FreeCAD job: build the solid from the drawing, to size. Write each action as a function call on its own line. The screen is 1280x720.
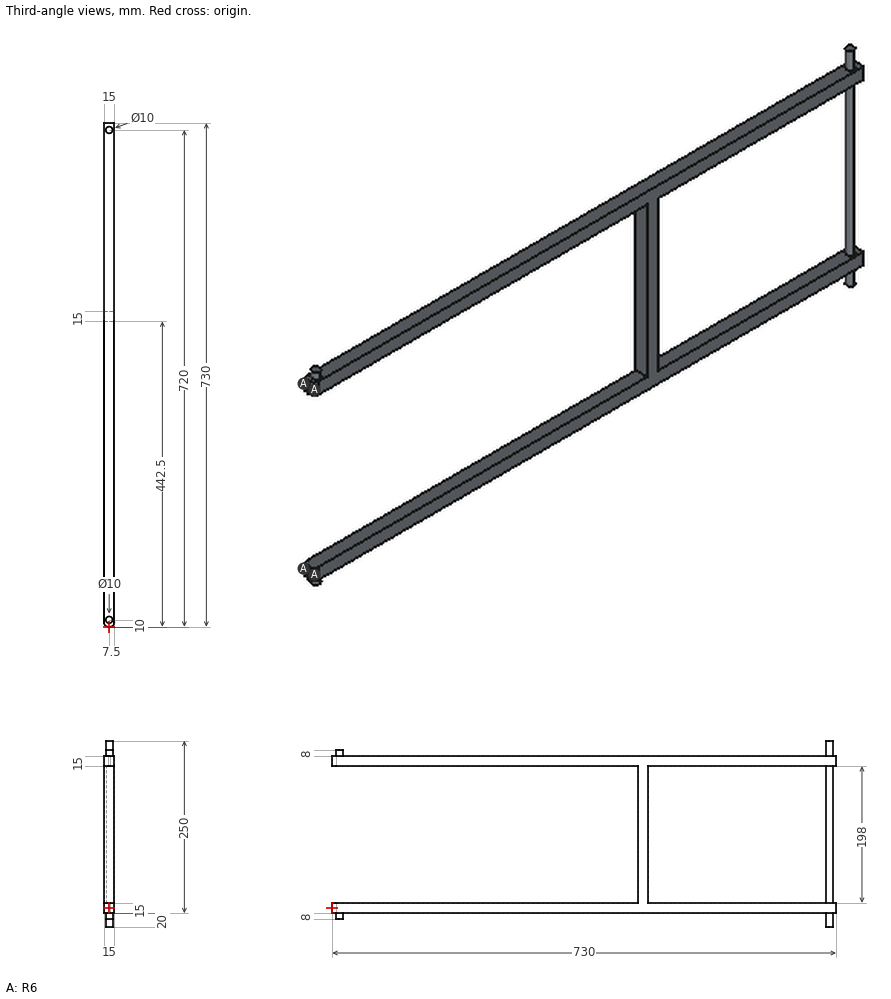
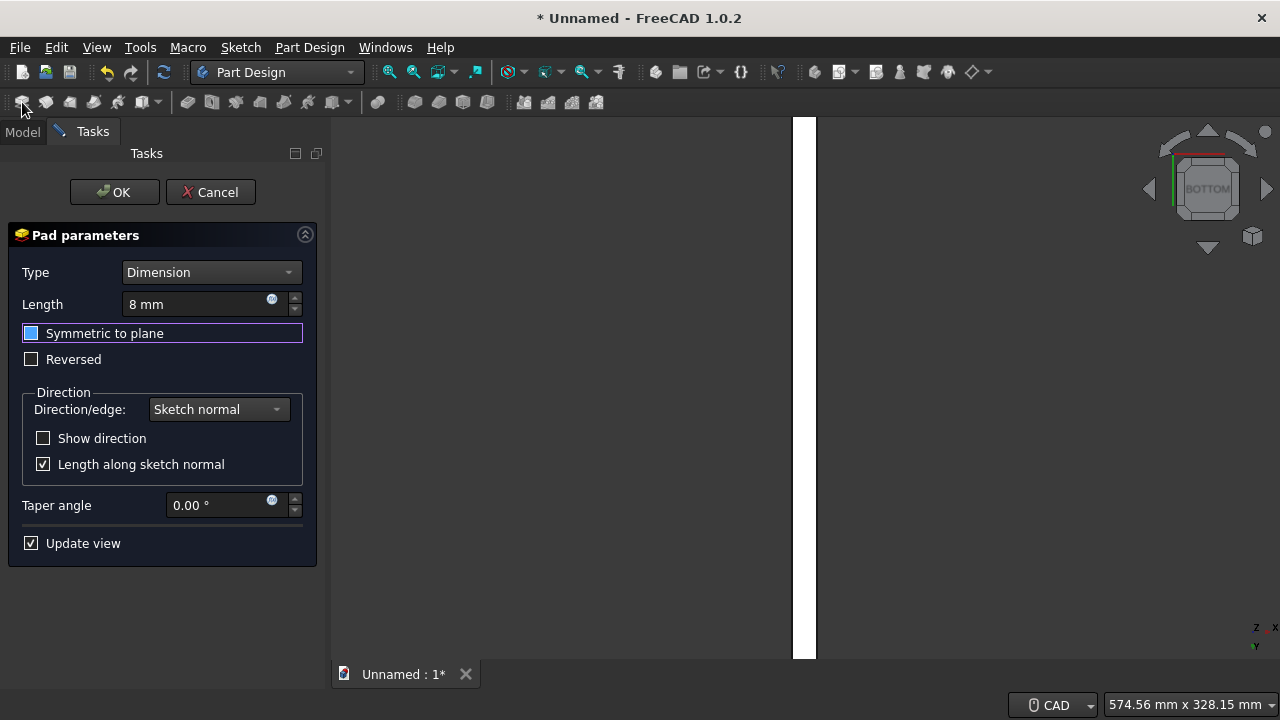
click(115, 192)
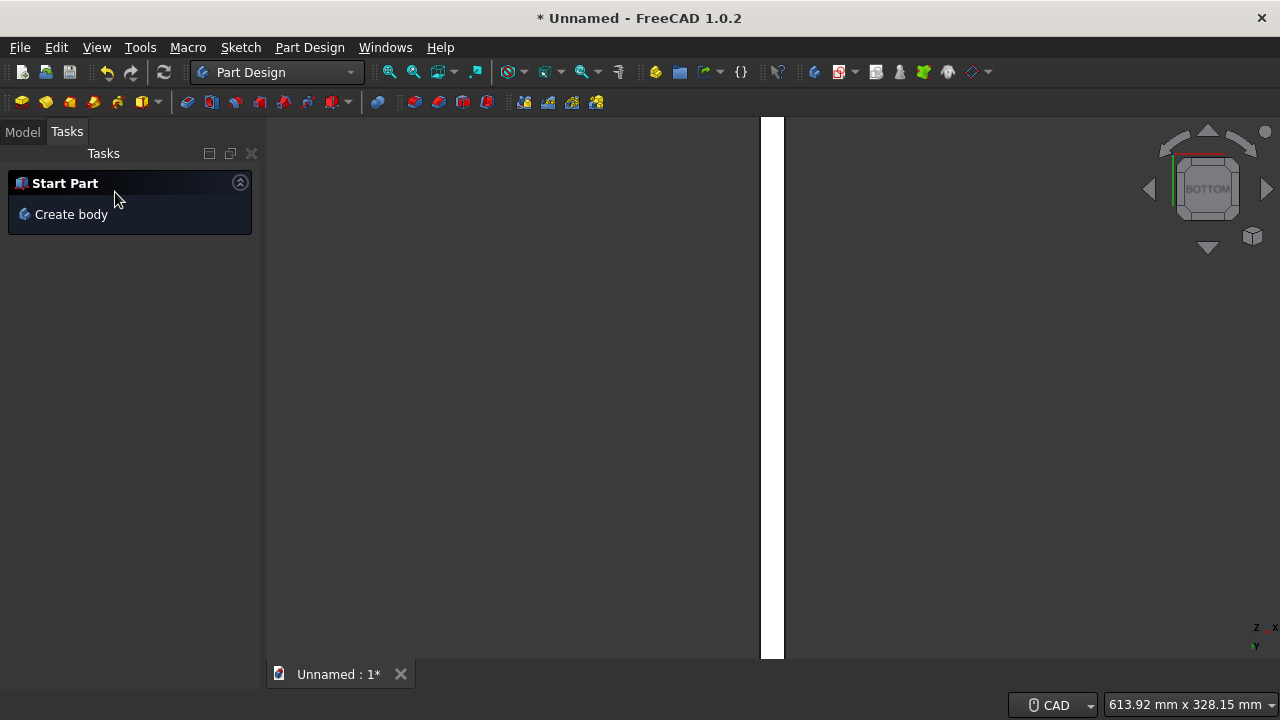
click(390, 72)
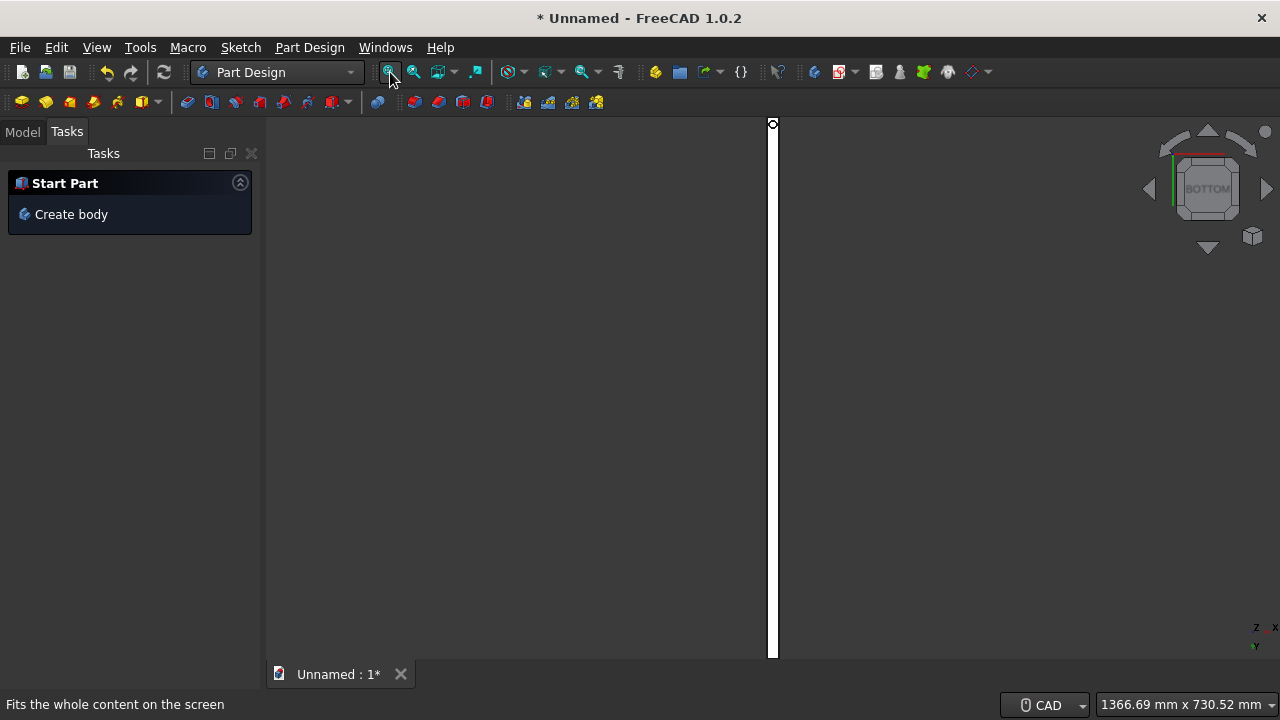
key(0)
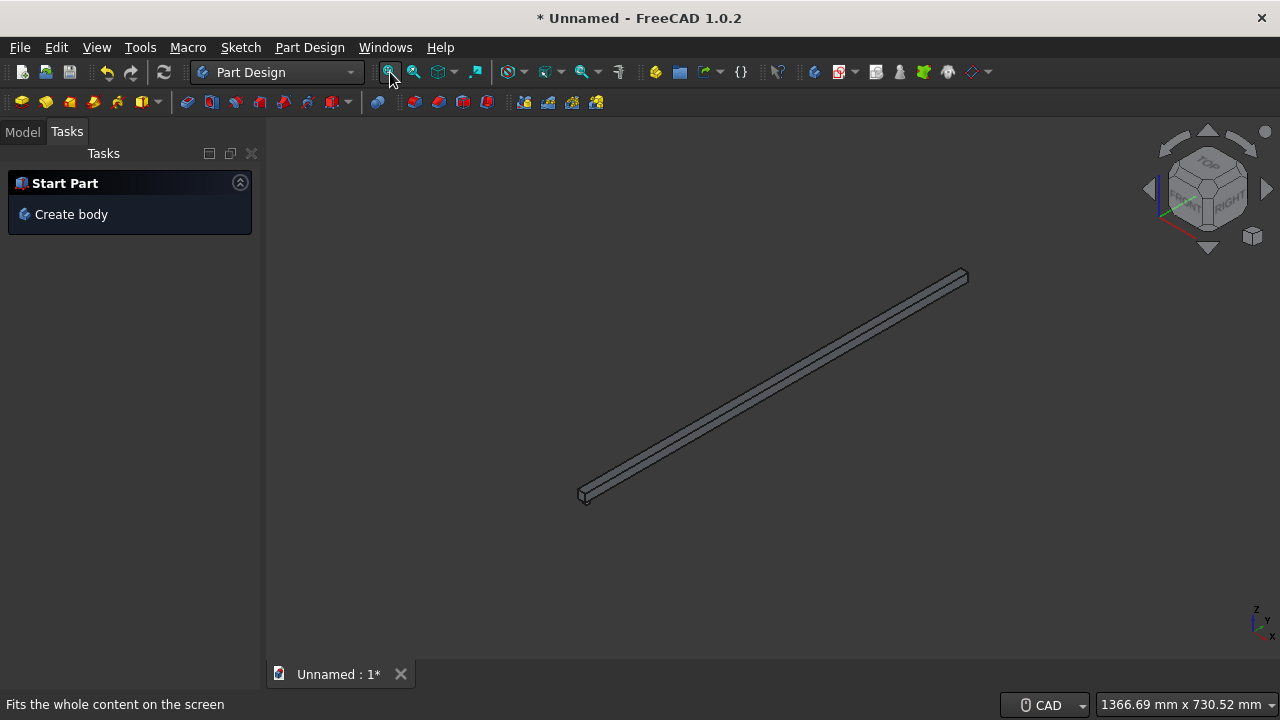
click(390, 72)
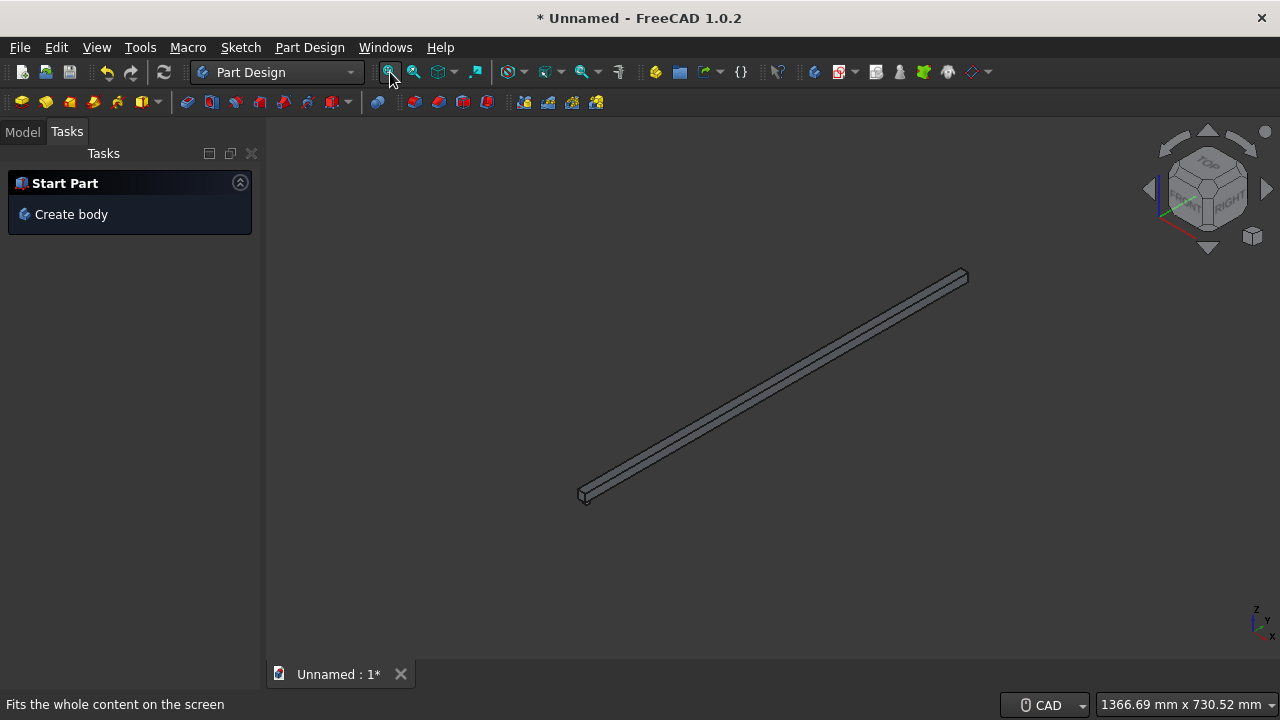
scroll(937, 285, up, 4)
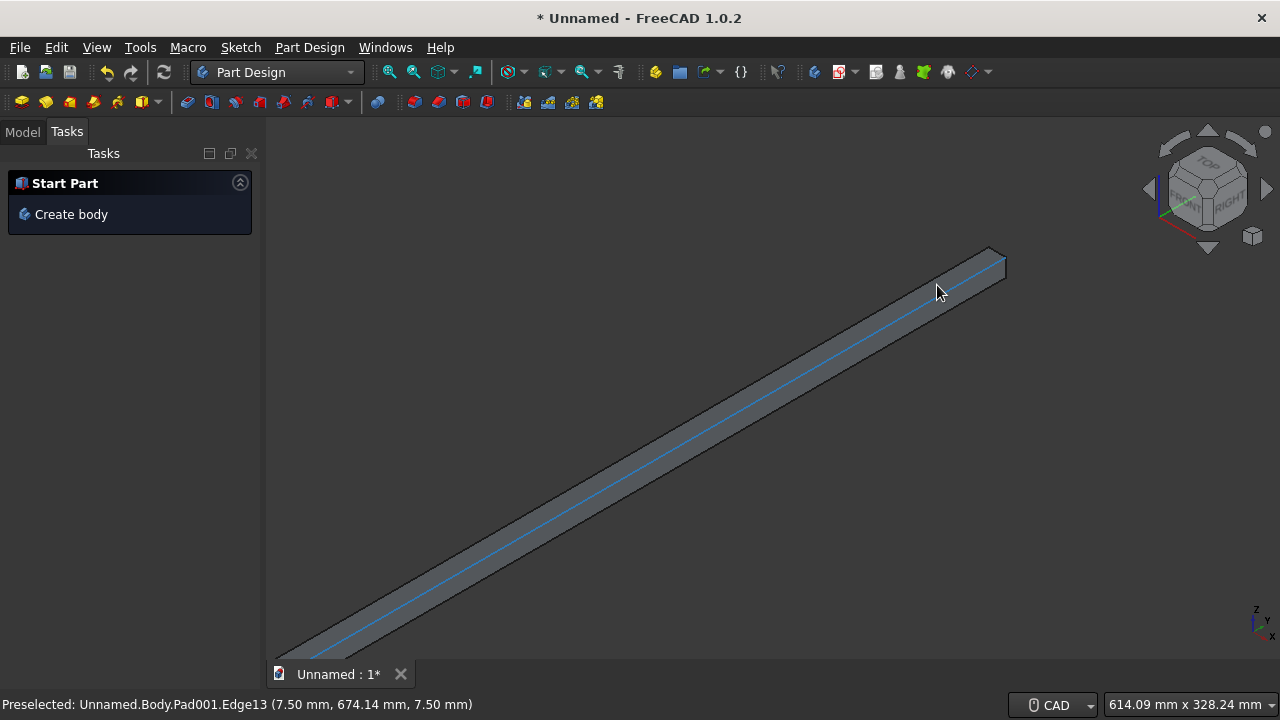
click(936, 286)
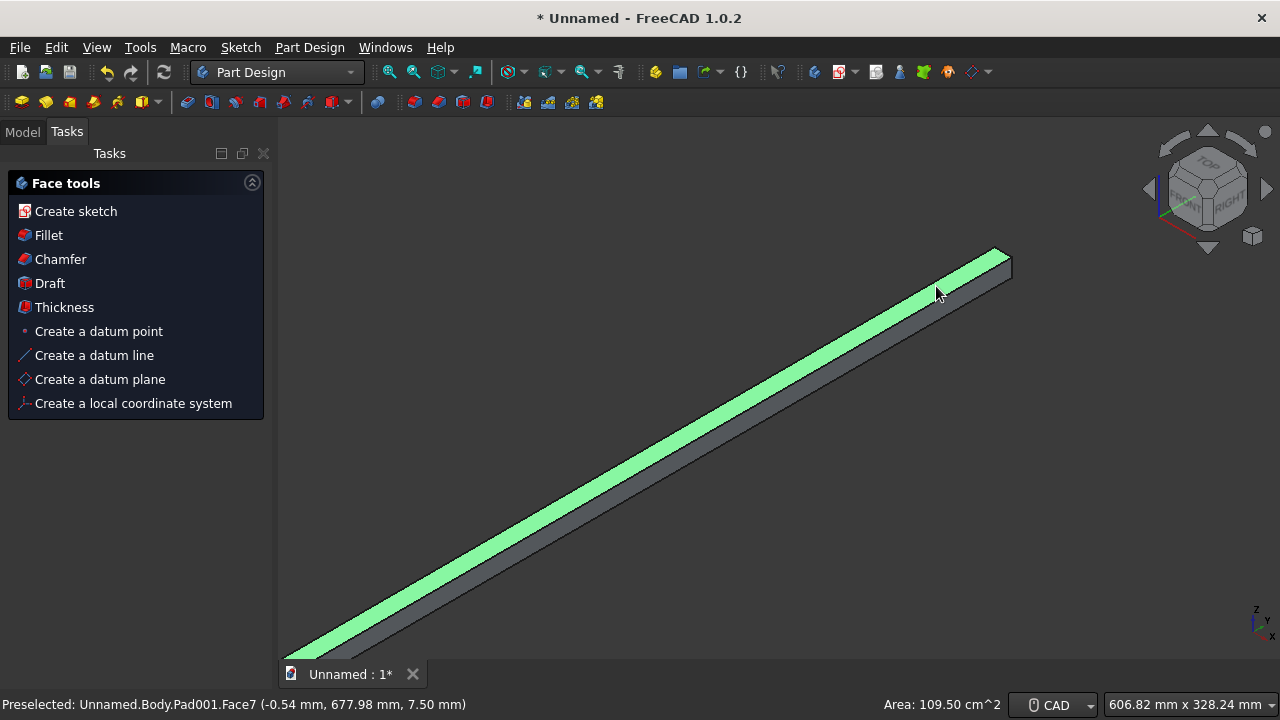
click(840, 72)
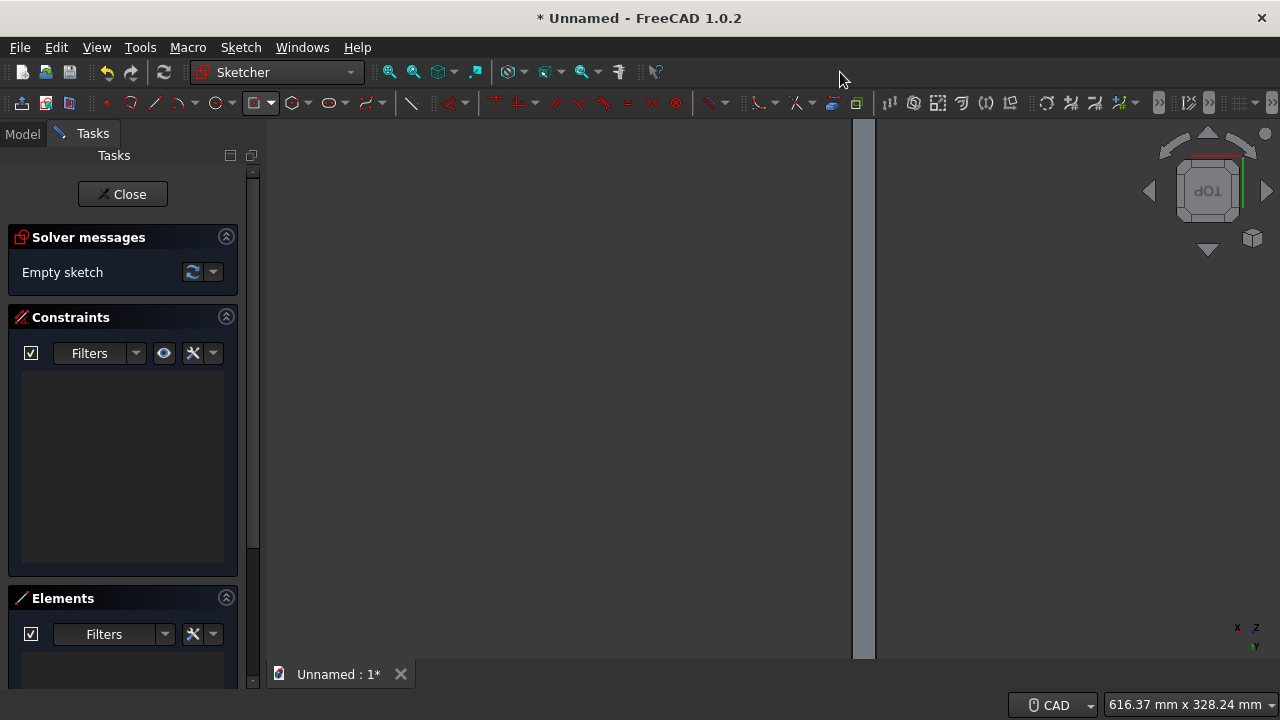
scroll(877, 331, up, 13)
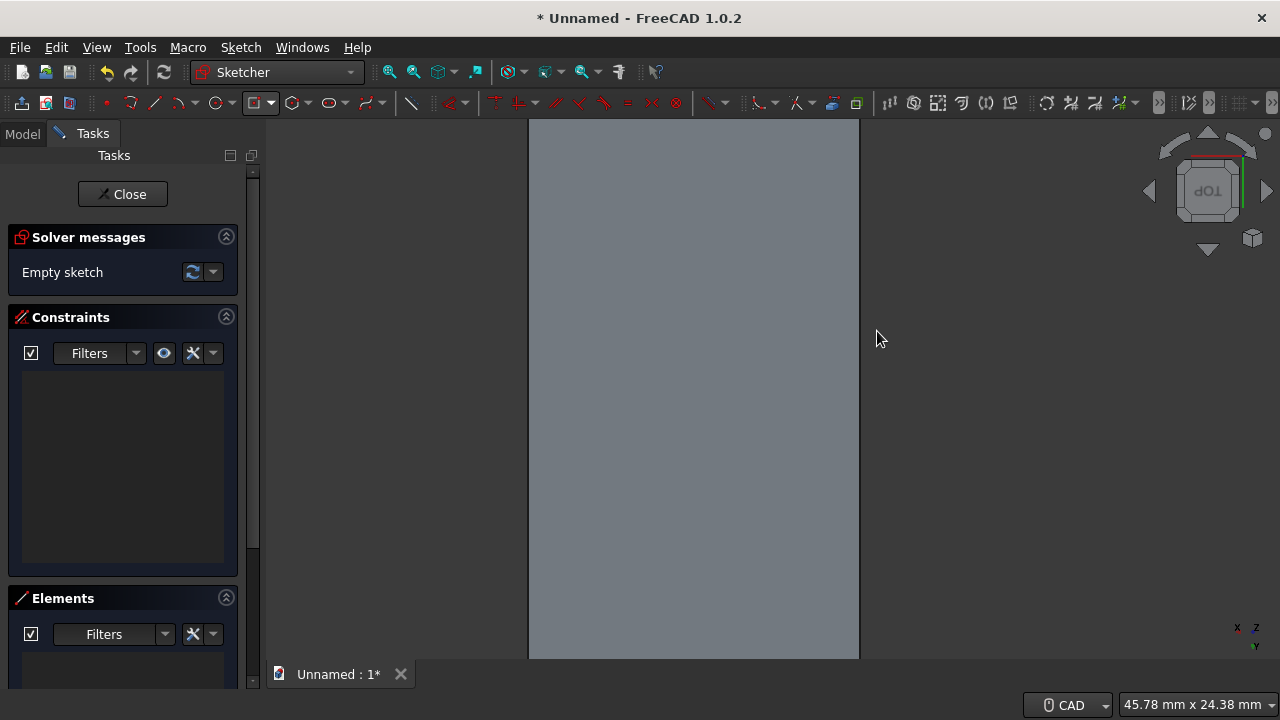
click(274, 104)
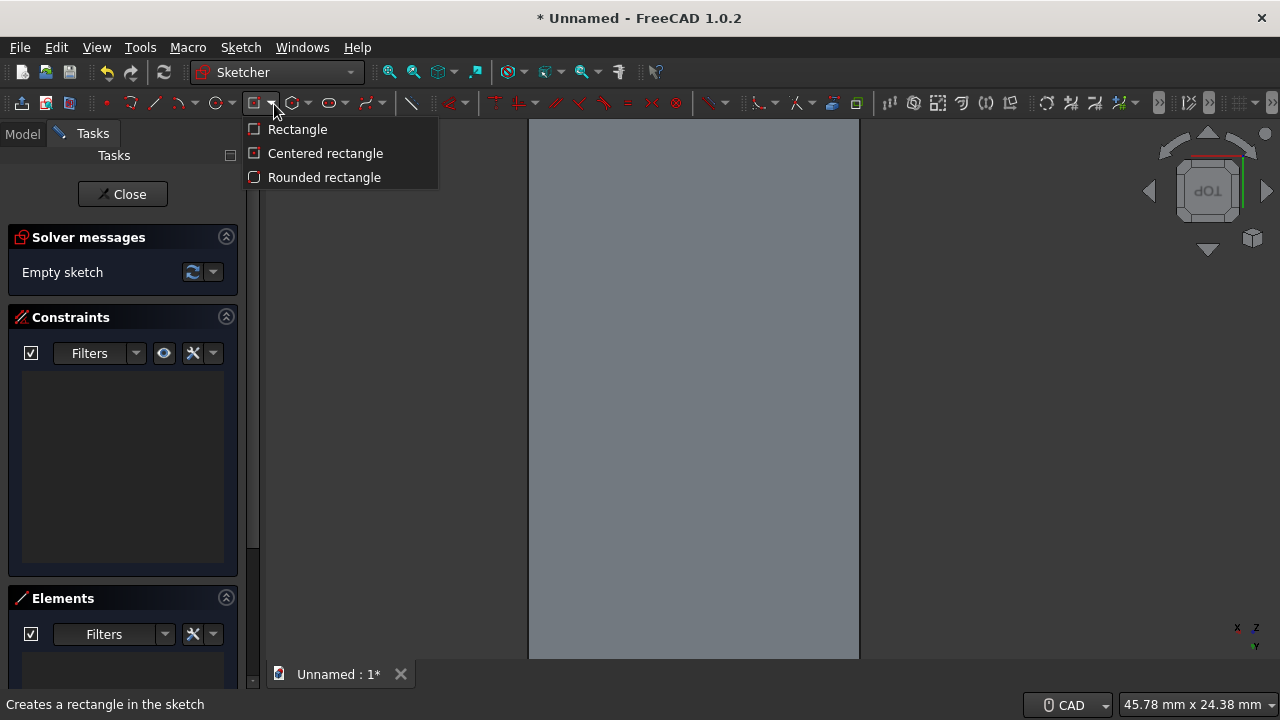
click(340, 129)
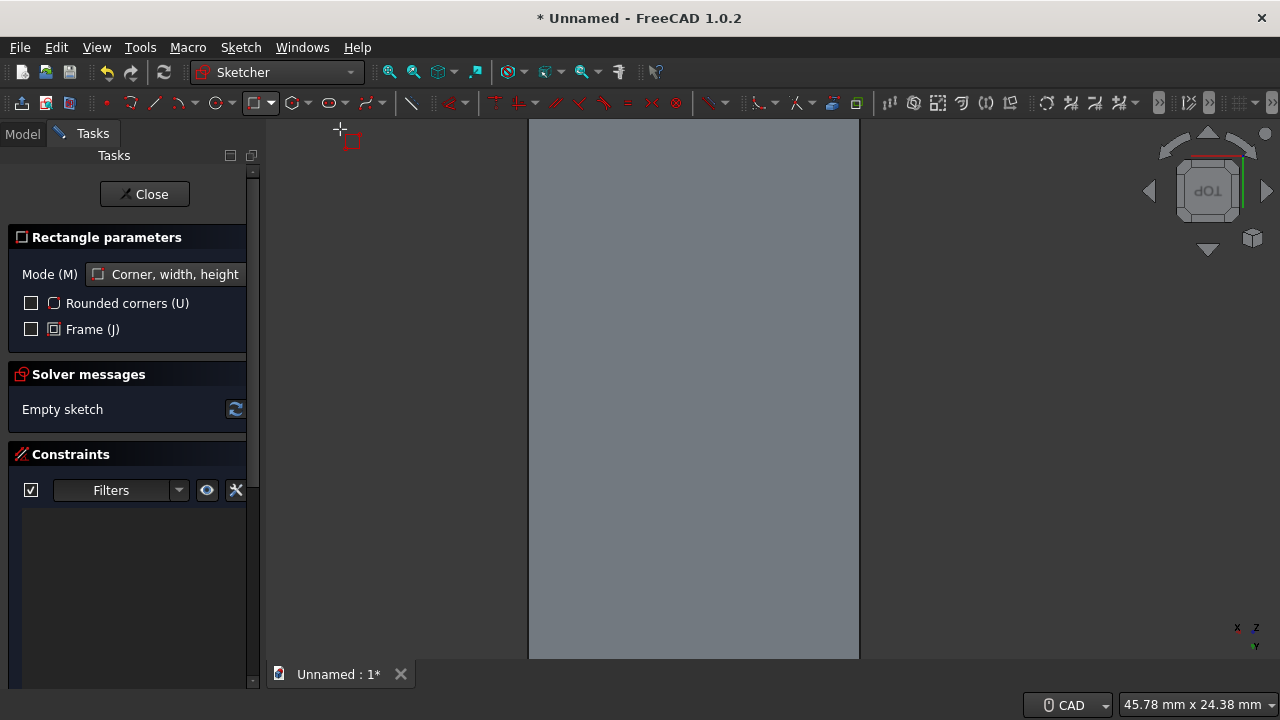
click(528, 220)
move(860, 553)